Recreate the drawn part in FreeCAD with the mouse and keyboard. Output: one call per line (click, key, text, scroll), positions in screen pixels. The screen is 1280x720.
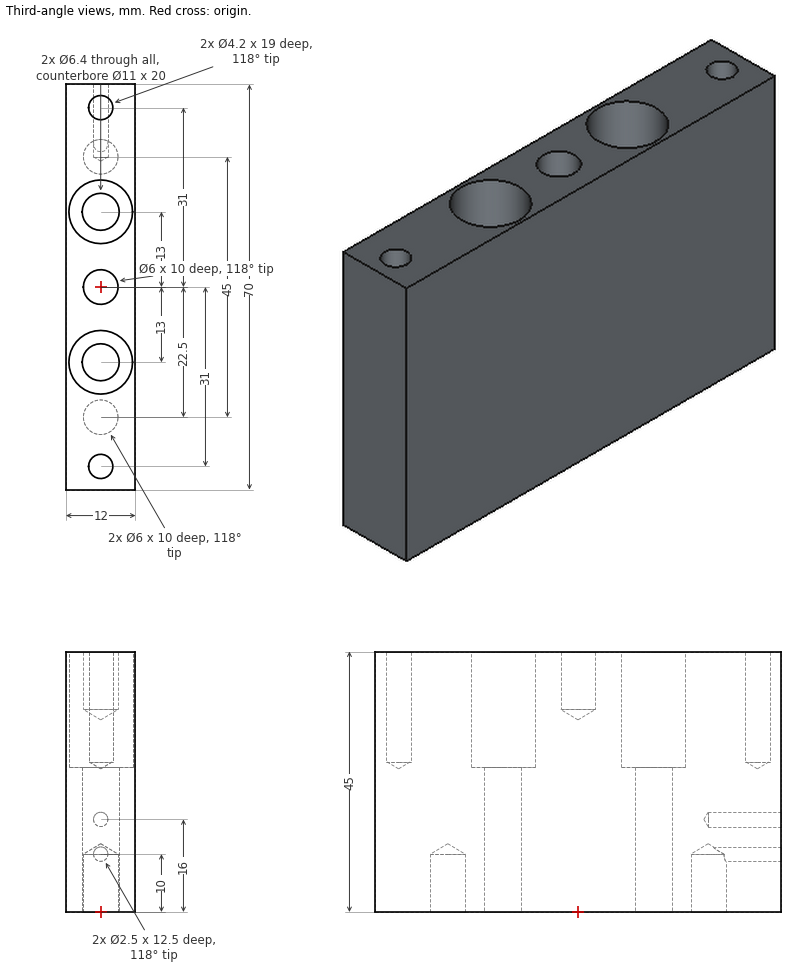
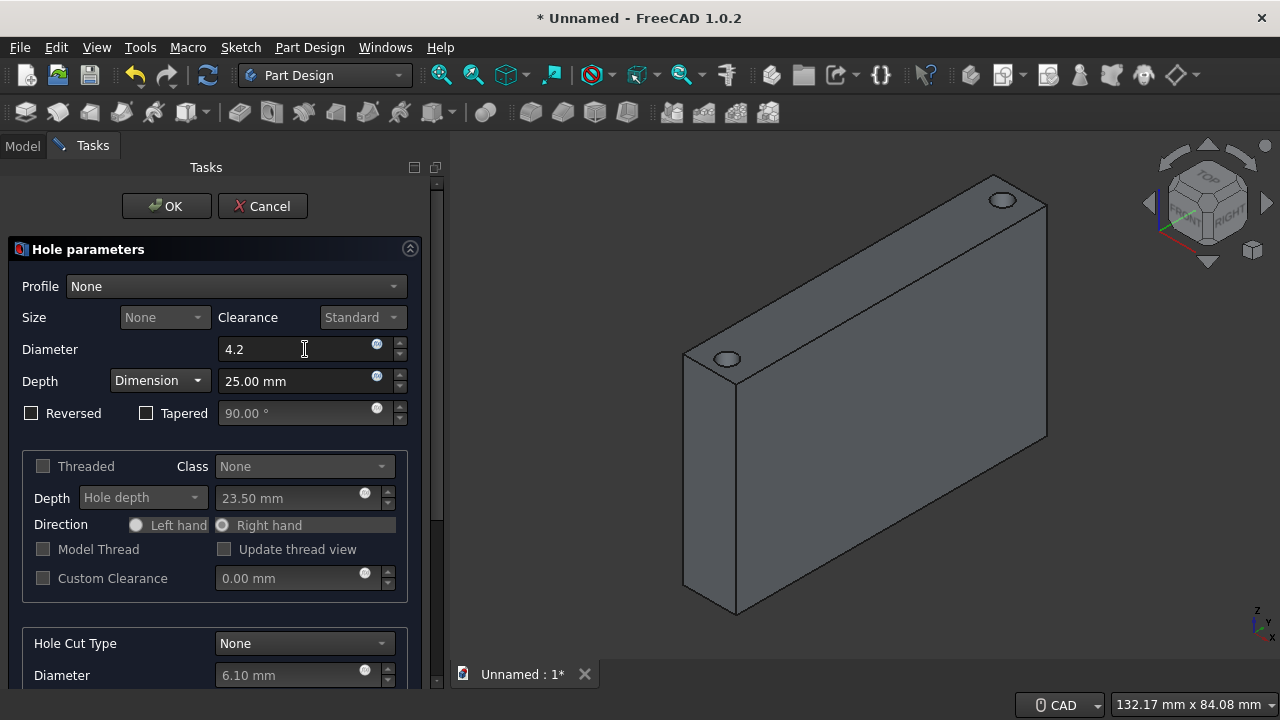
triple_click(305, 381)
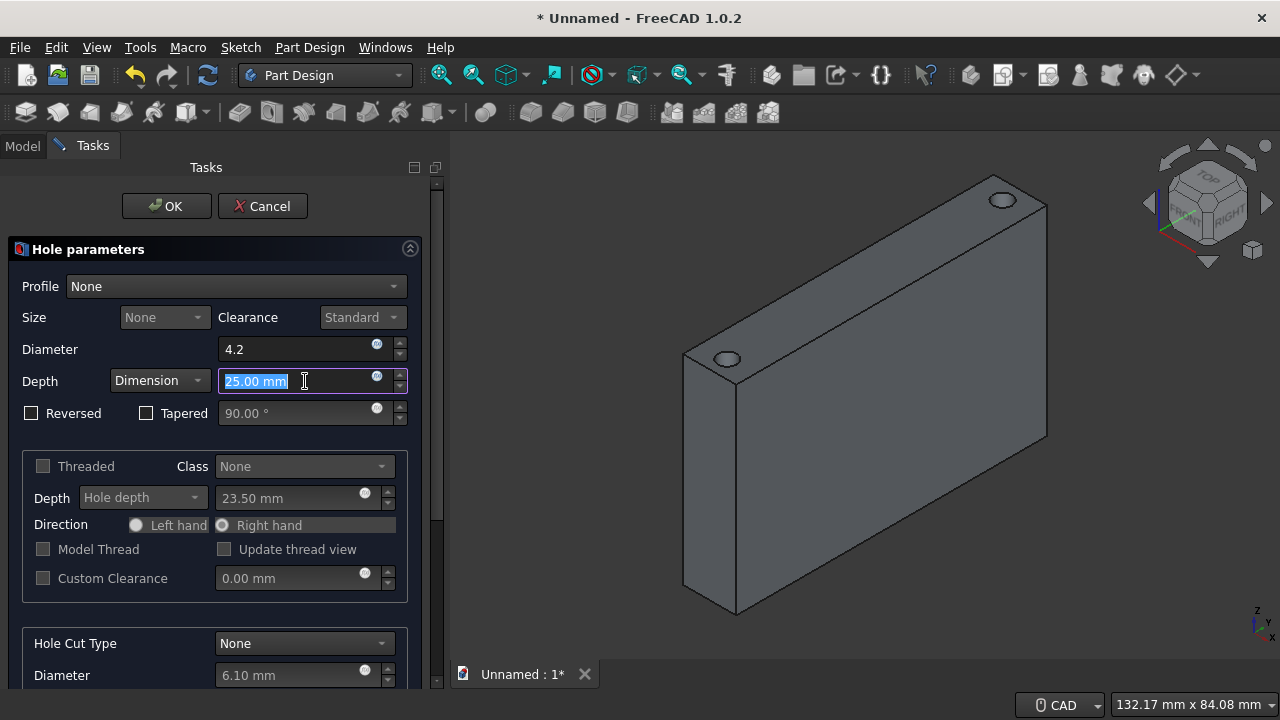
text(19)
key(Tab)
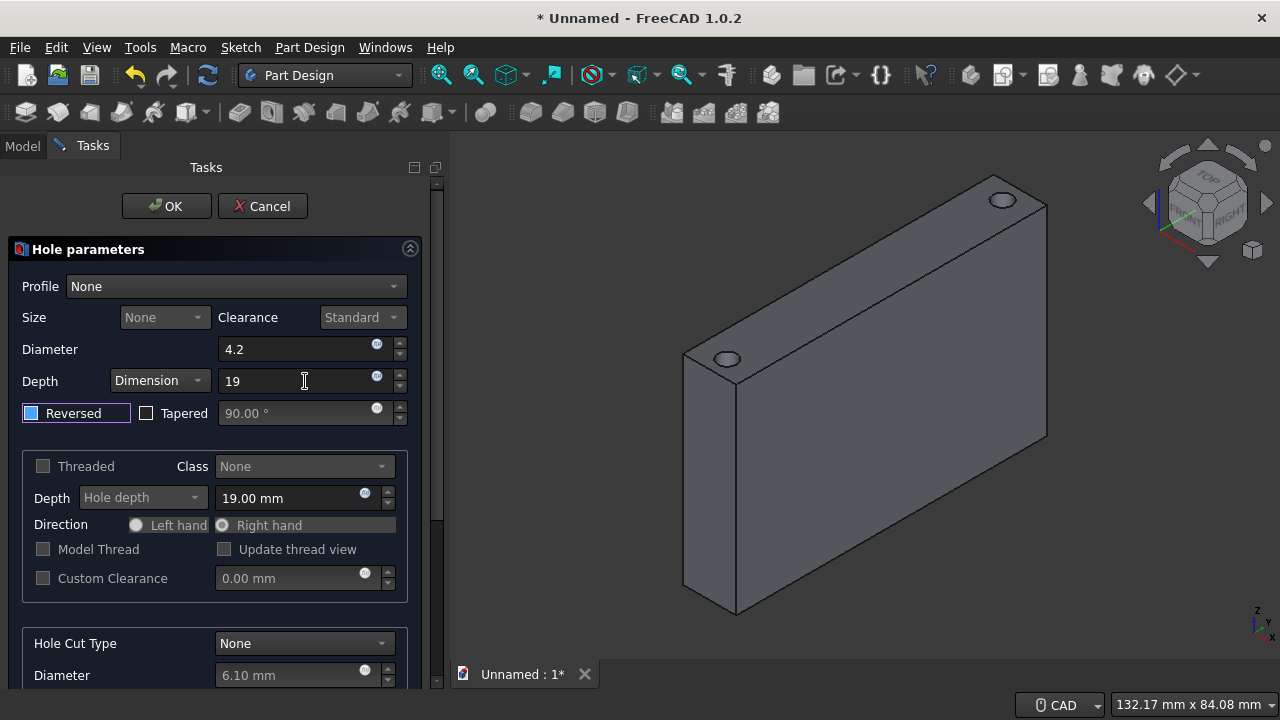
click(167, 206)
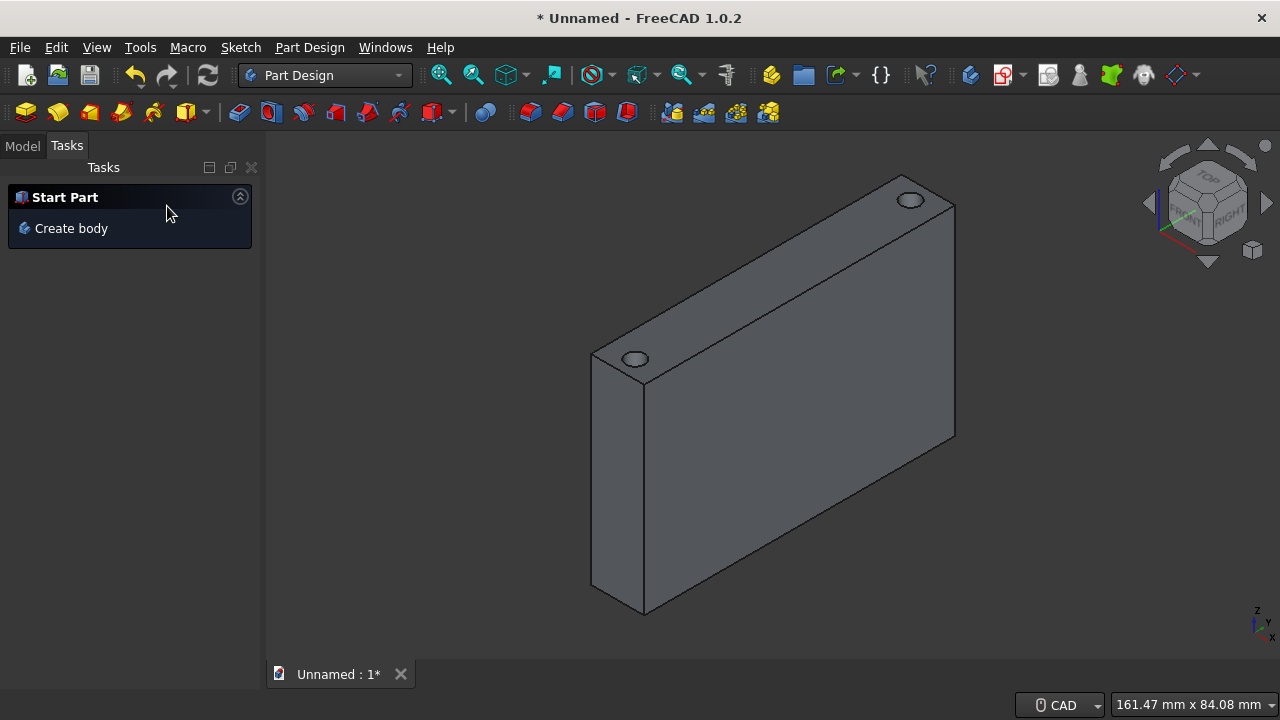
click(862, 227)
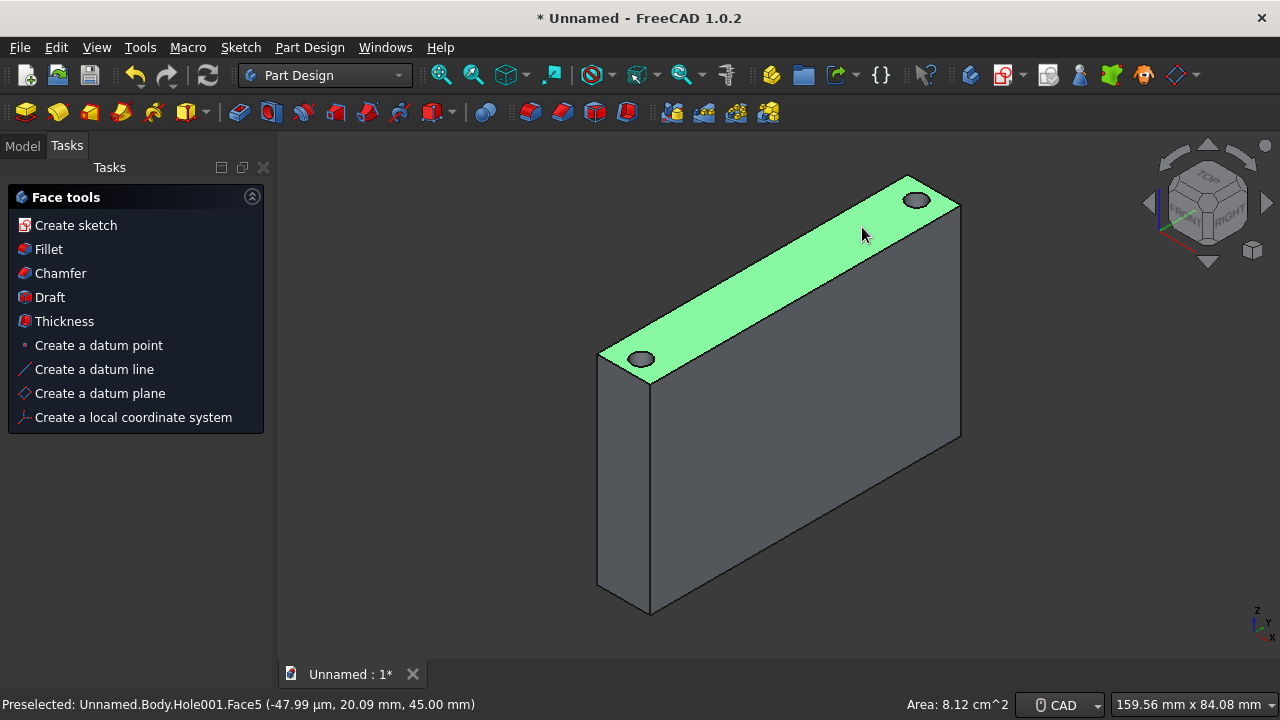
click(1004, 76)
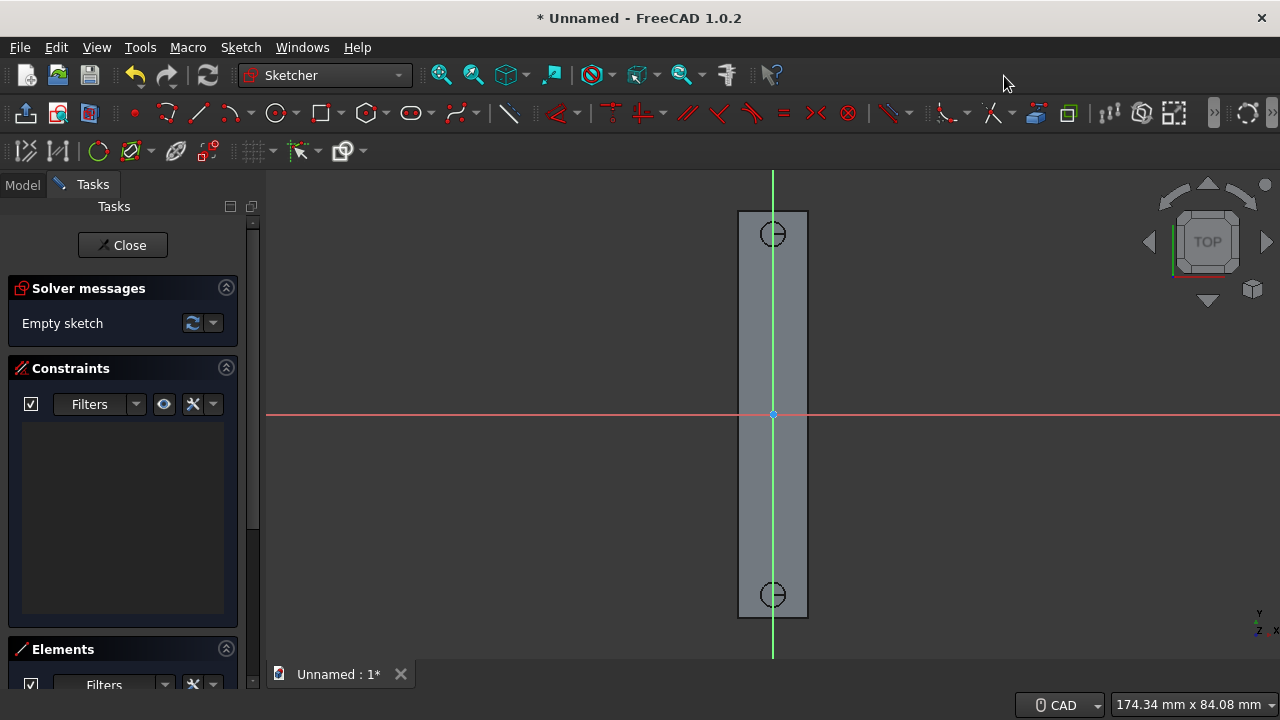
scroll(912, 414, up, 2)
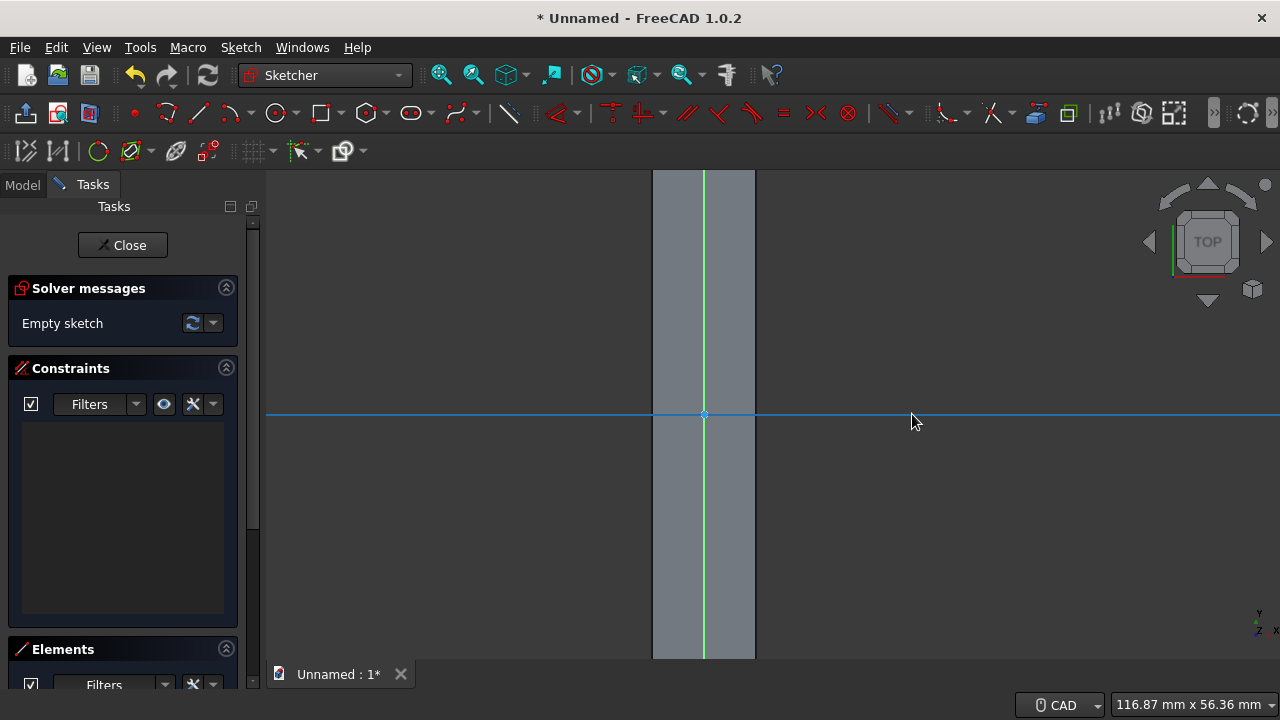
click(276, 114)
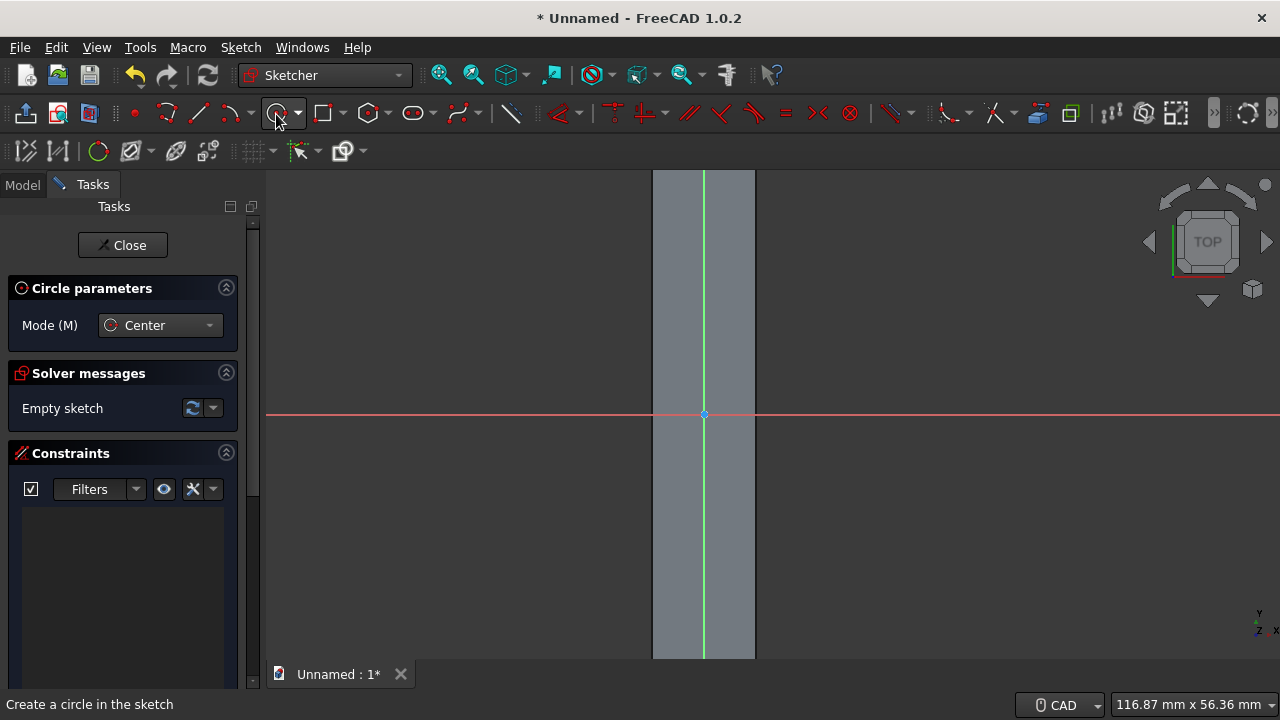
click(704, 302)
move(724, 282)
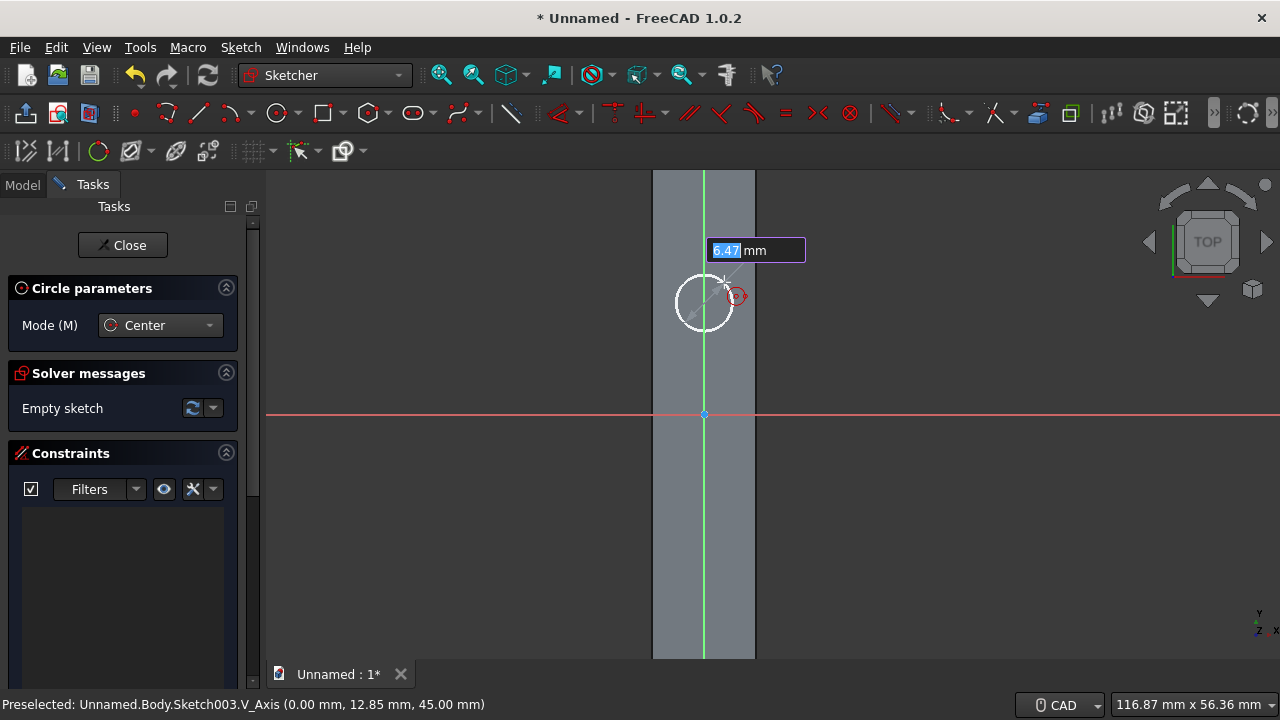
text(6.4)
key(Return)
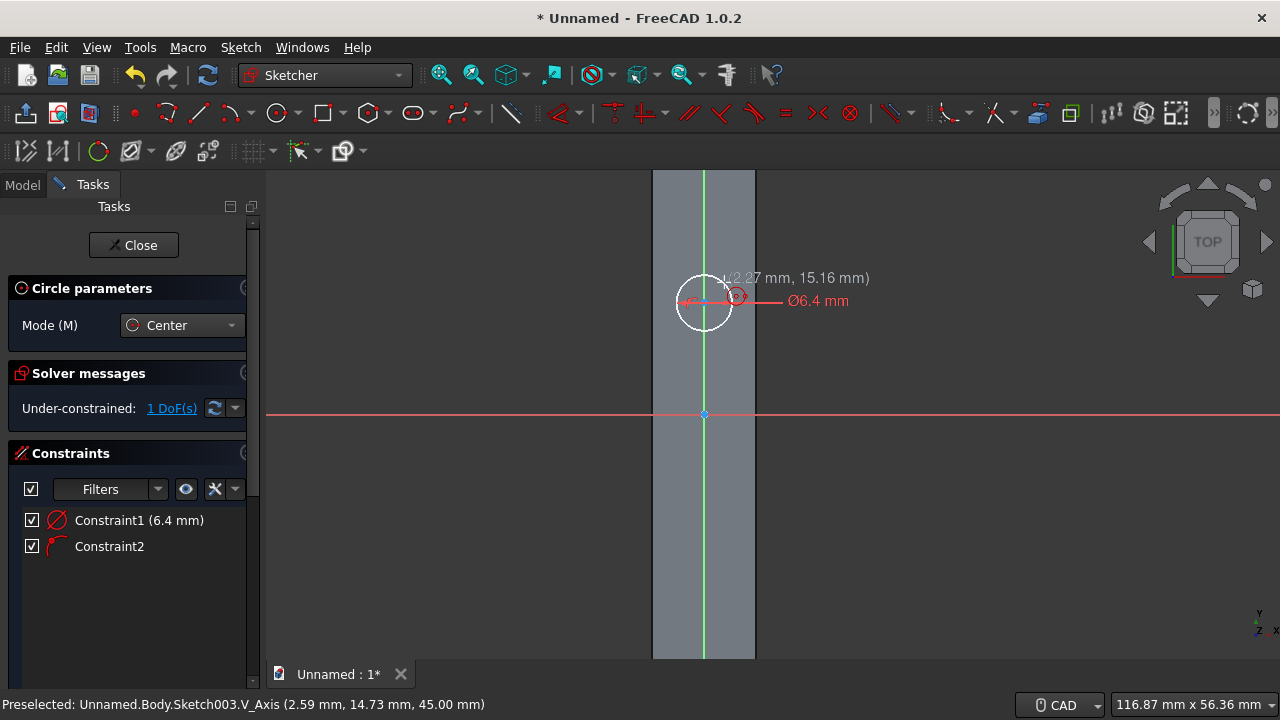
click(704, 527)
move(724, 508)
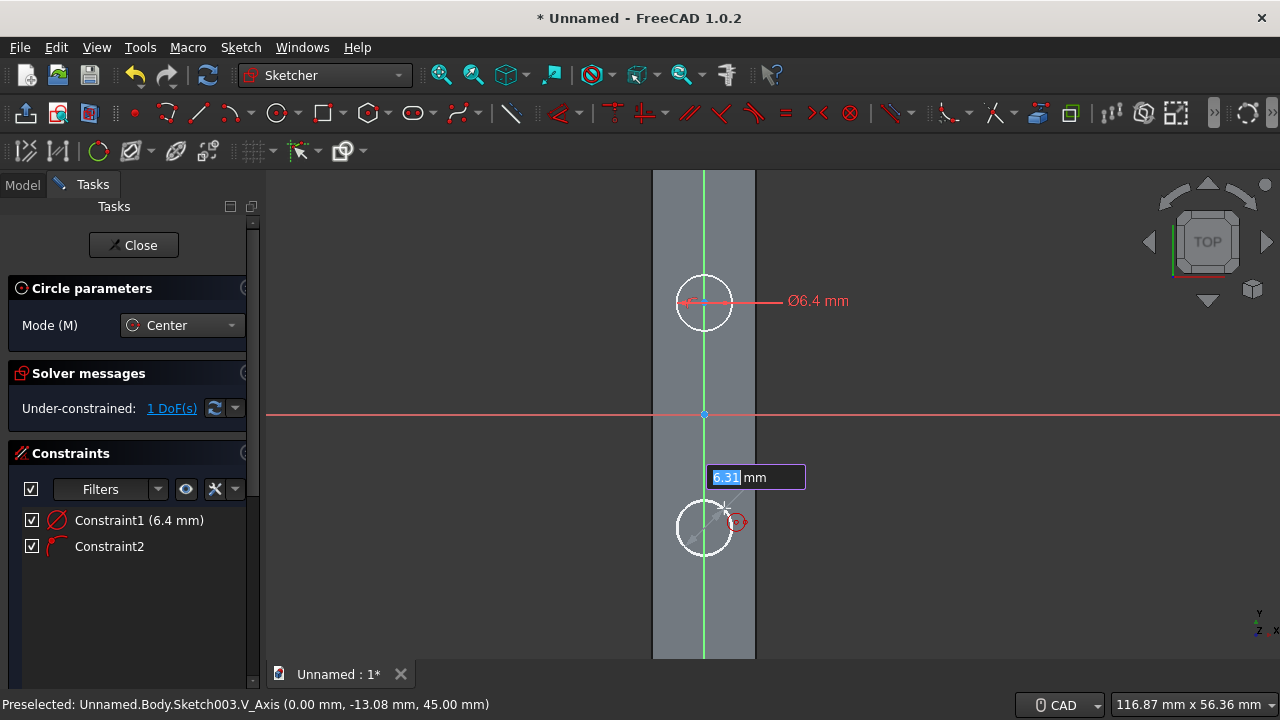
text(6.4)
key(Return)
key(Escape)